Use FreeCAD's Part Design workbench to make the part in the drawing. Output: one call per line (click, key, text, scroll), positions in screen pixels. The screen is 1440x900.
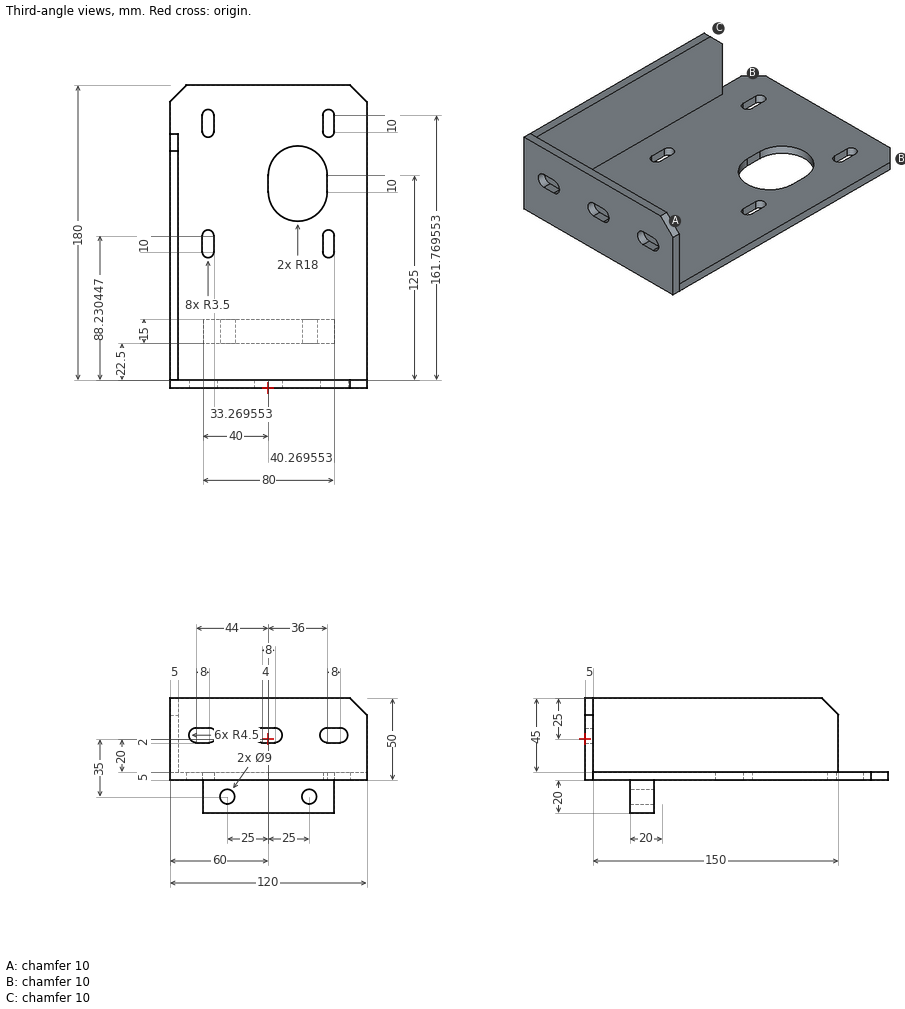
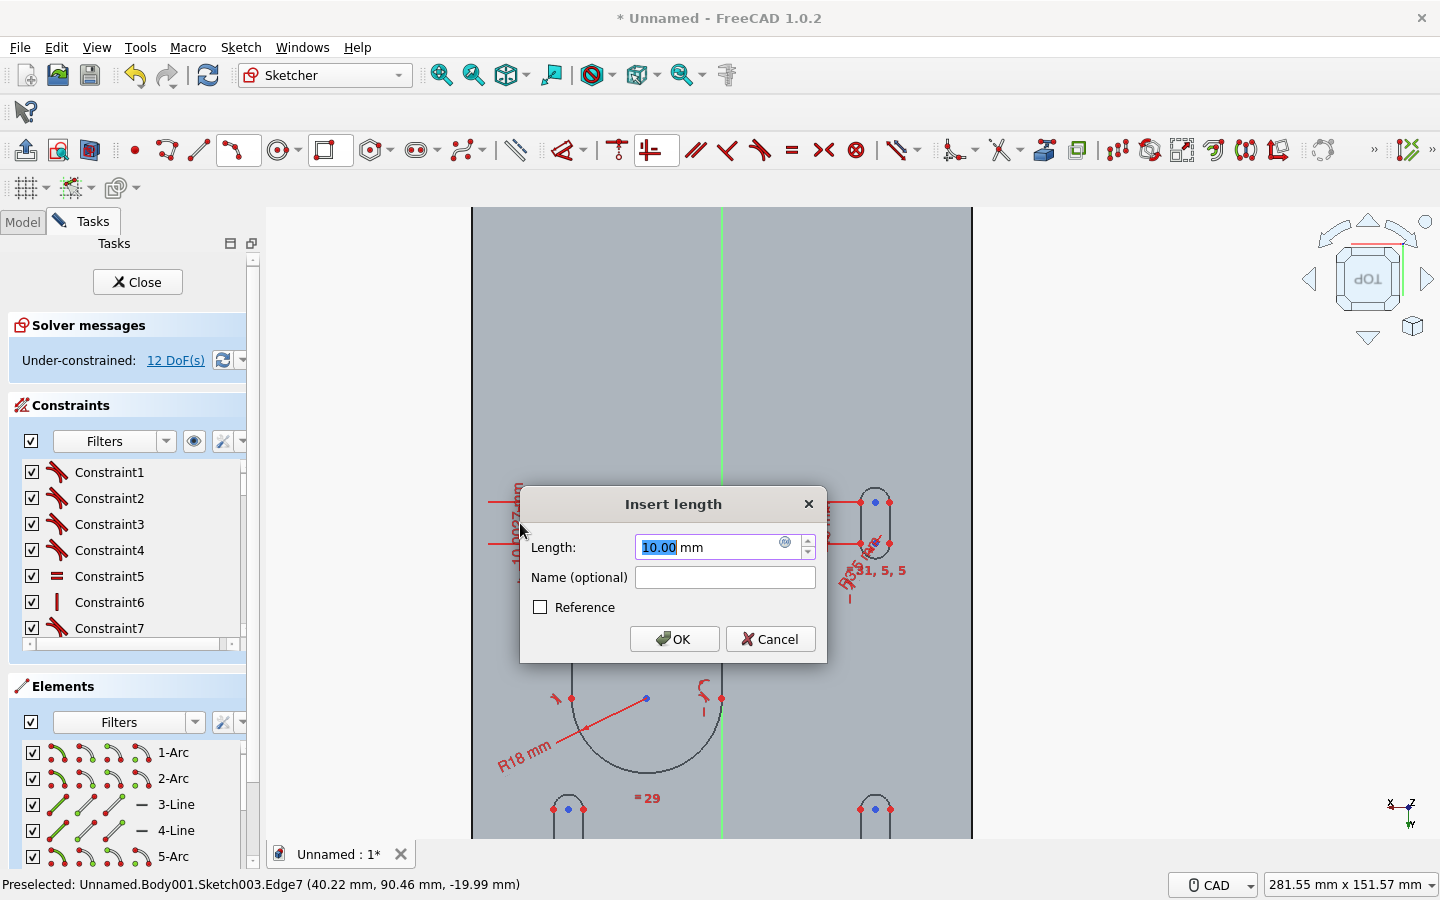
text(10)
key(Return)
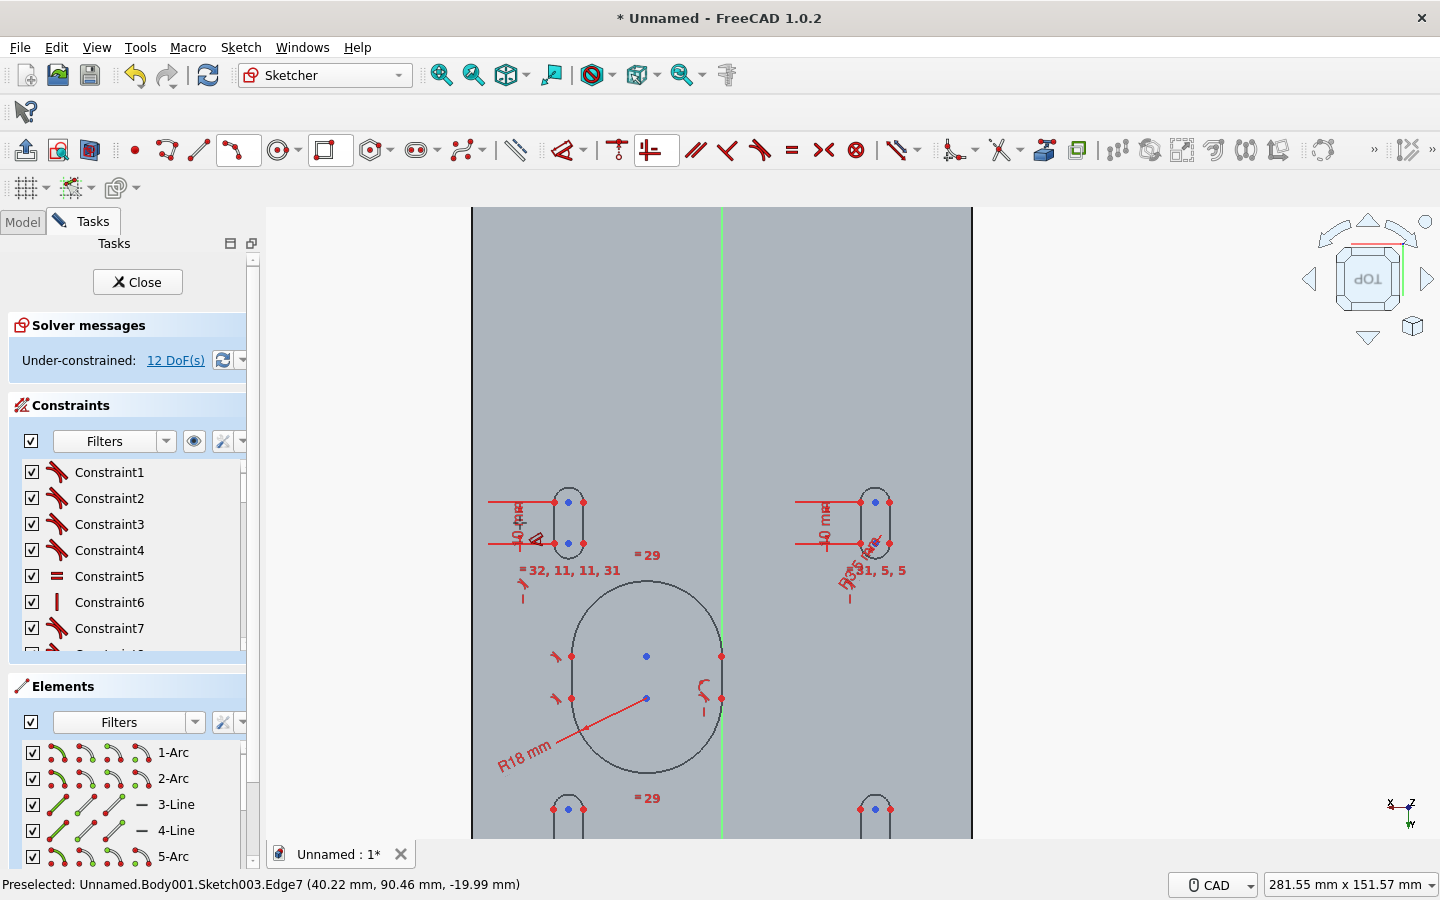
scroll(861, 526, down, 3)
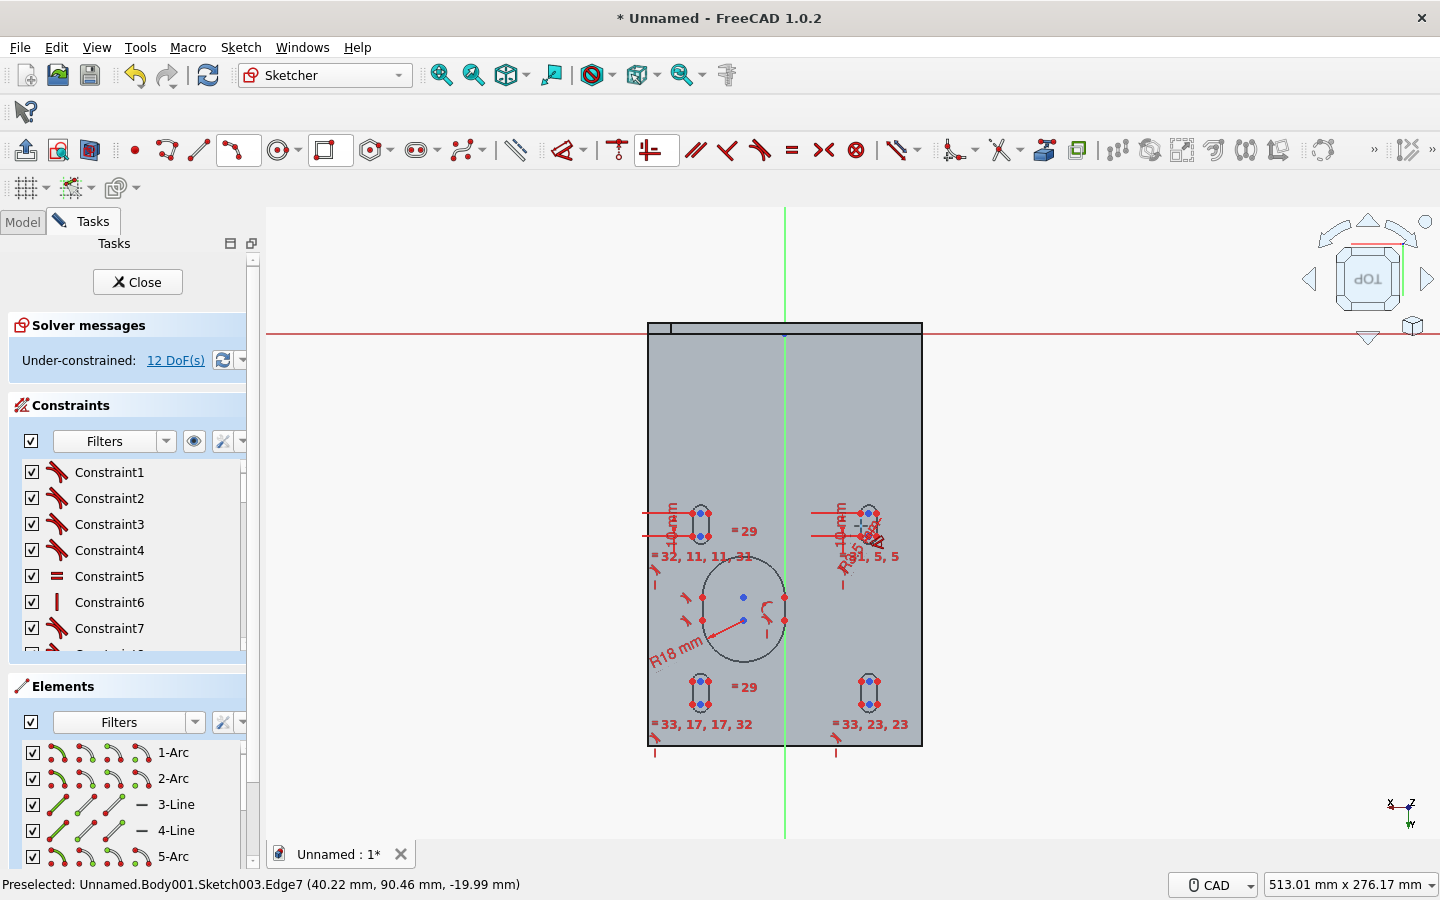
scroll(693, 698, up, 4)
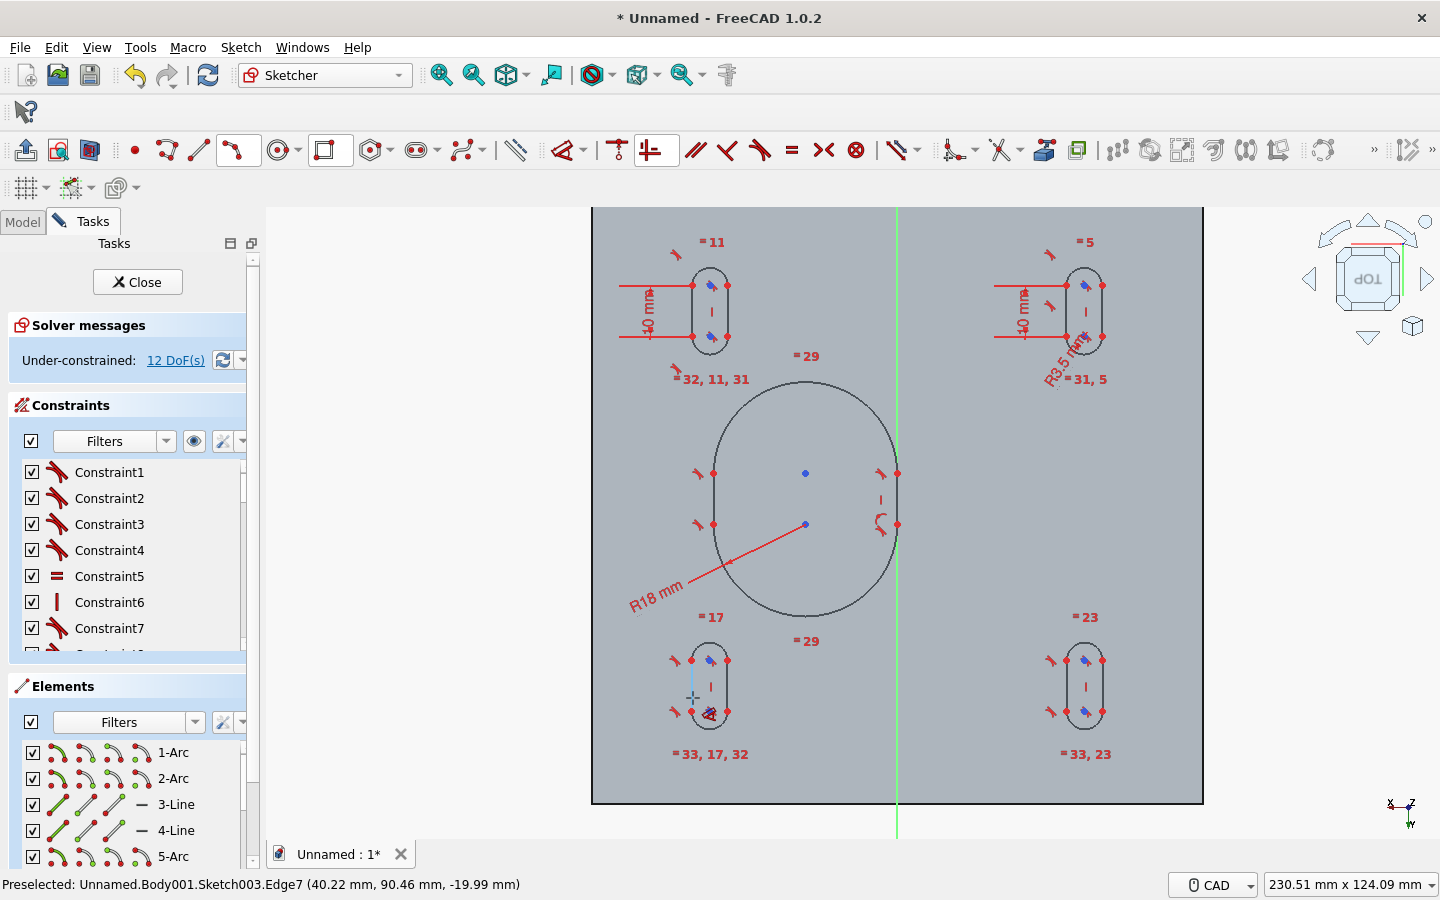
click(692, 696)
click(658, 686)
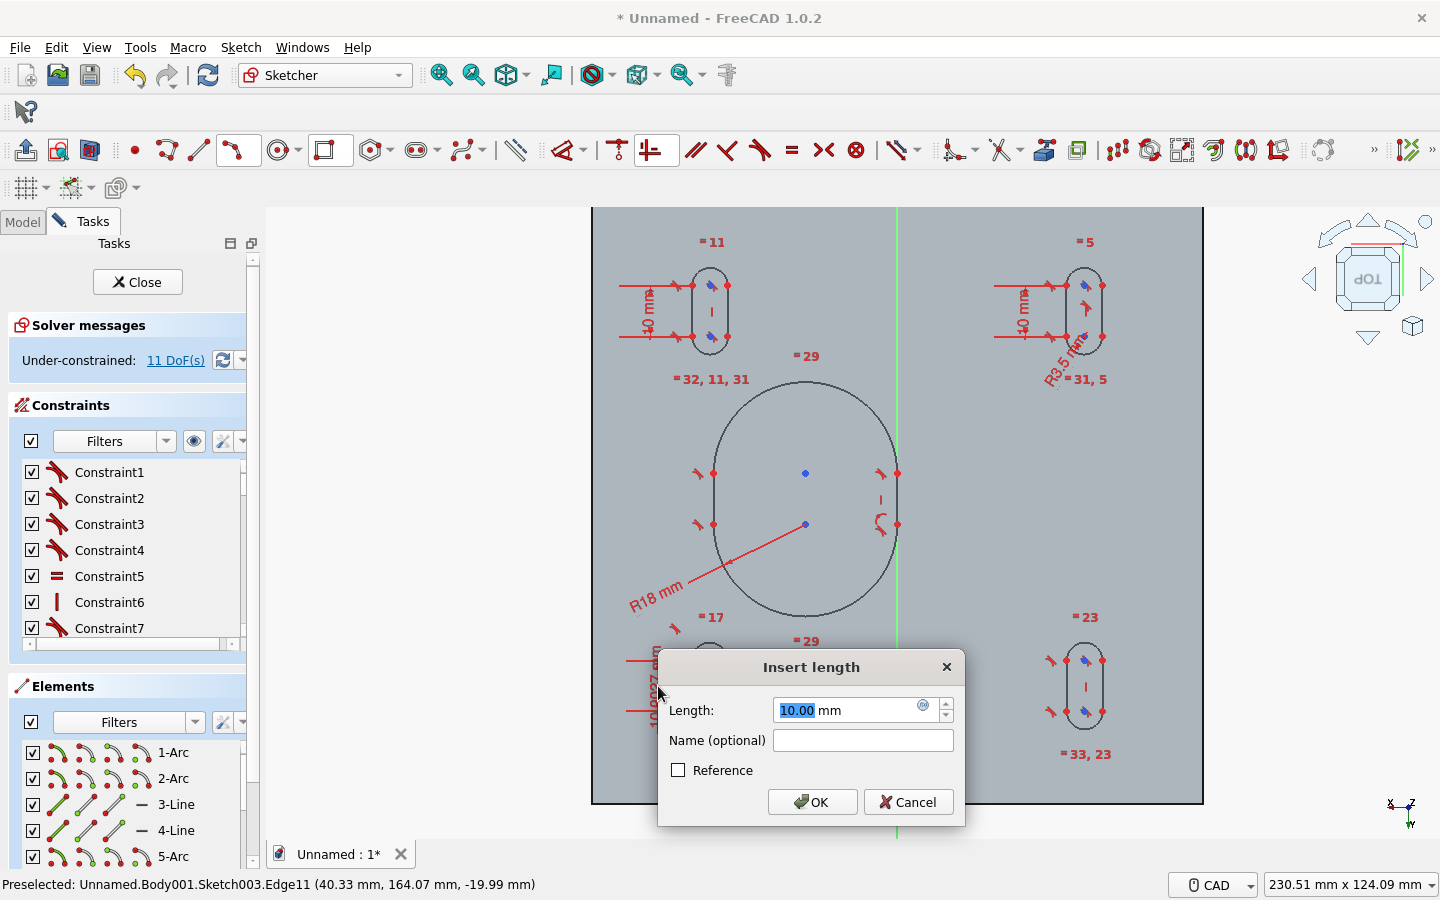
text(10)
key(Return)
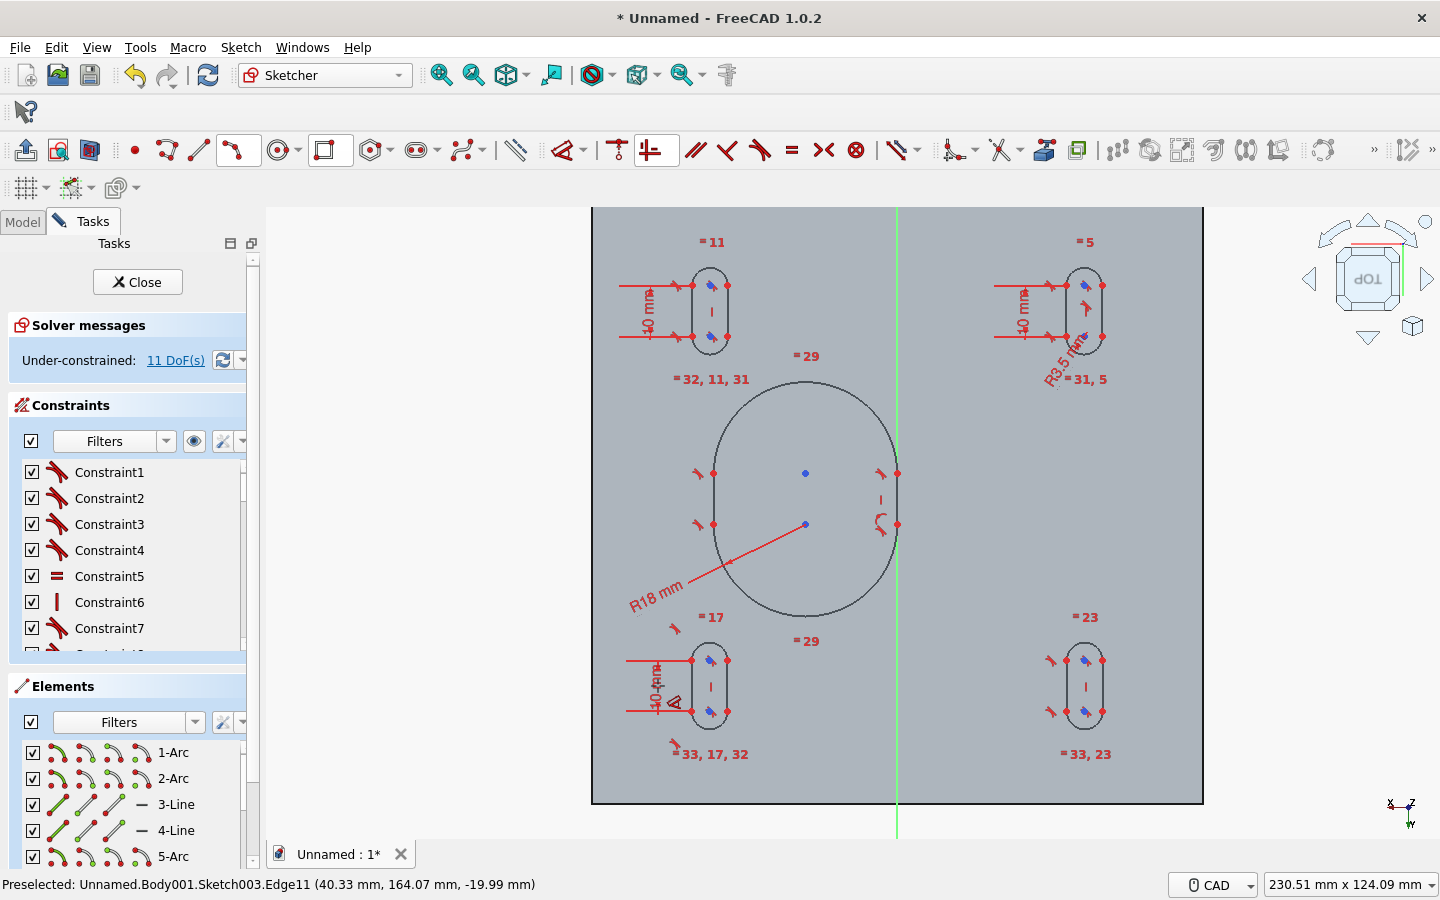
click(1067, 696)
click(1033, 686)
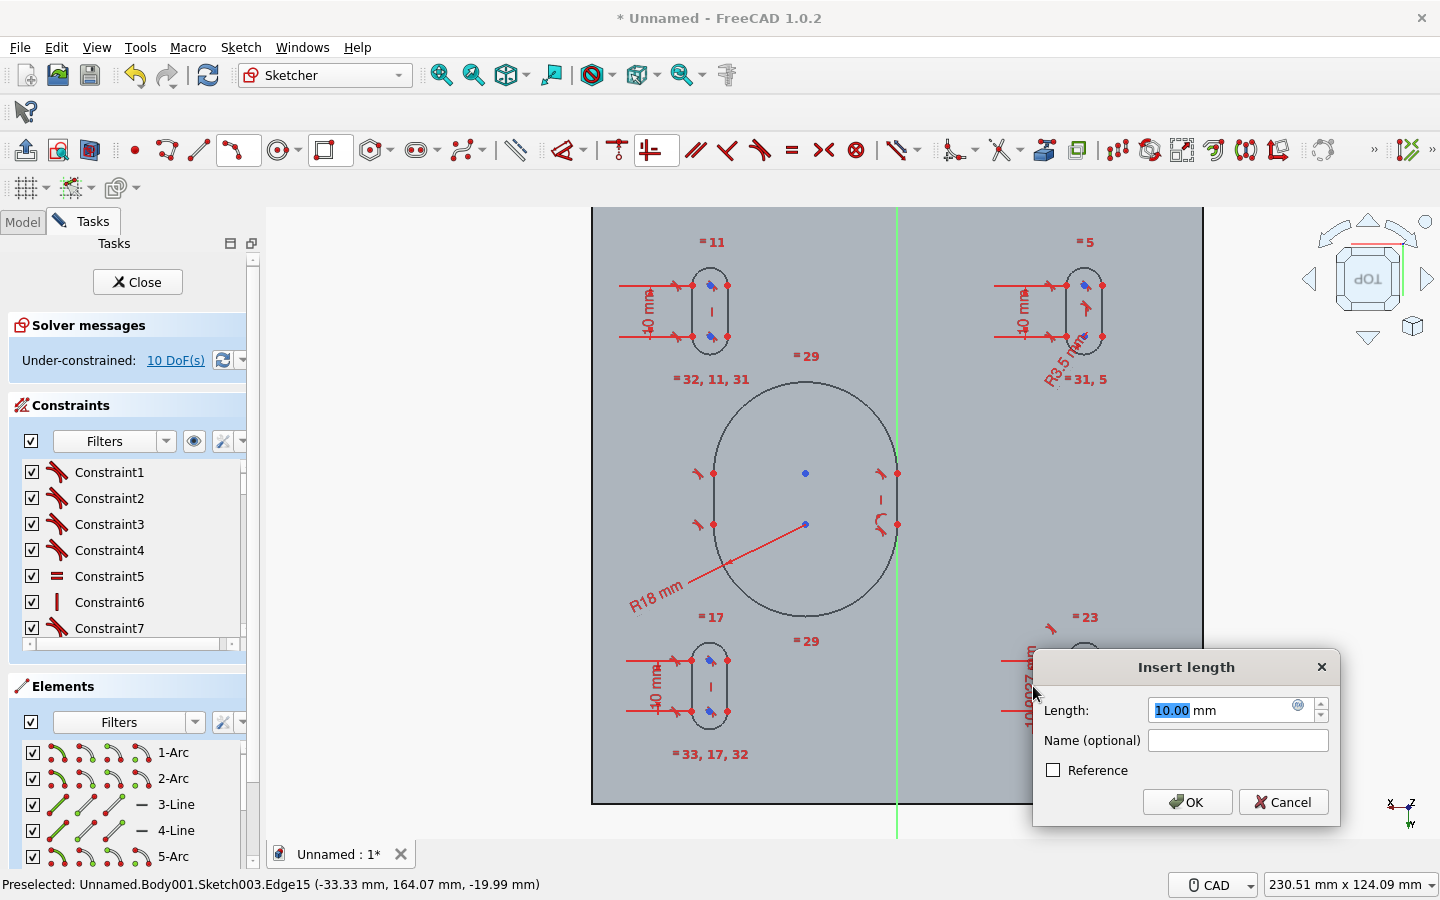
text(10)
key(Return)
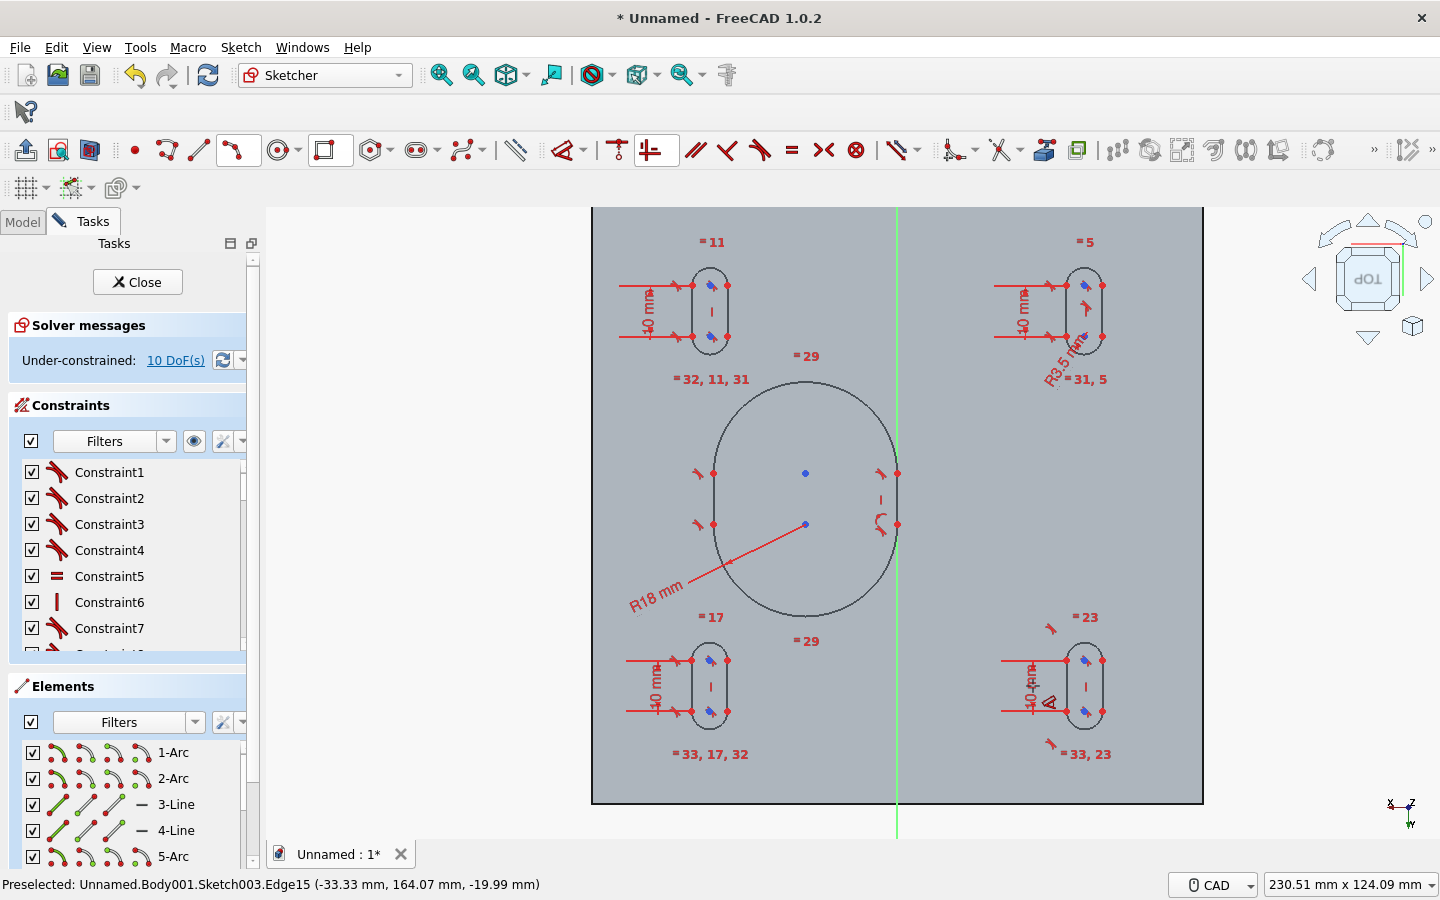
click(714, 510)
click(680, 499)